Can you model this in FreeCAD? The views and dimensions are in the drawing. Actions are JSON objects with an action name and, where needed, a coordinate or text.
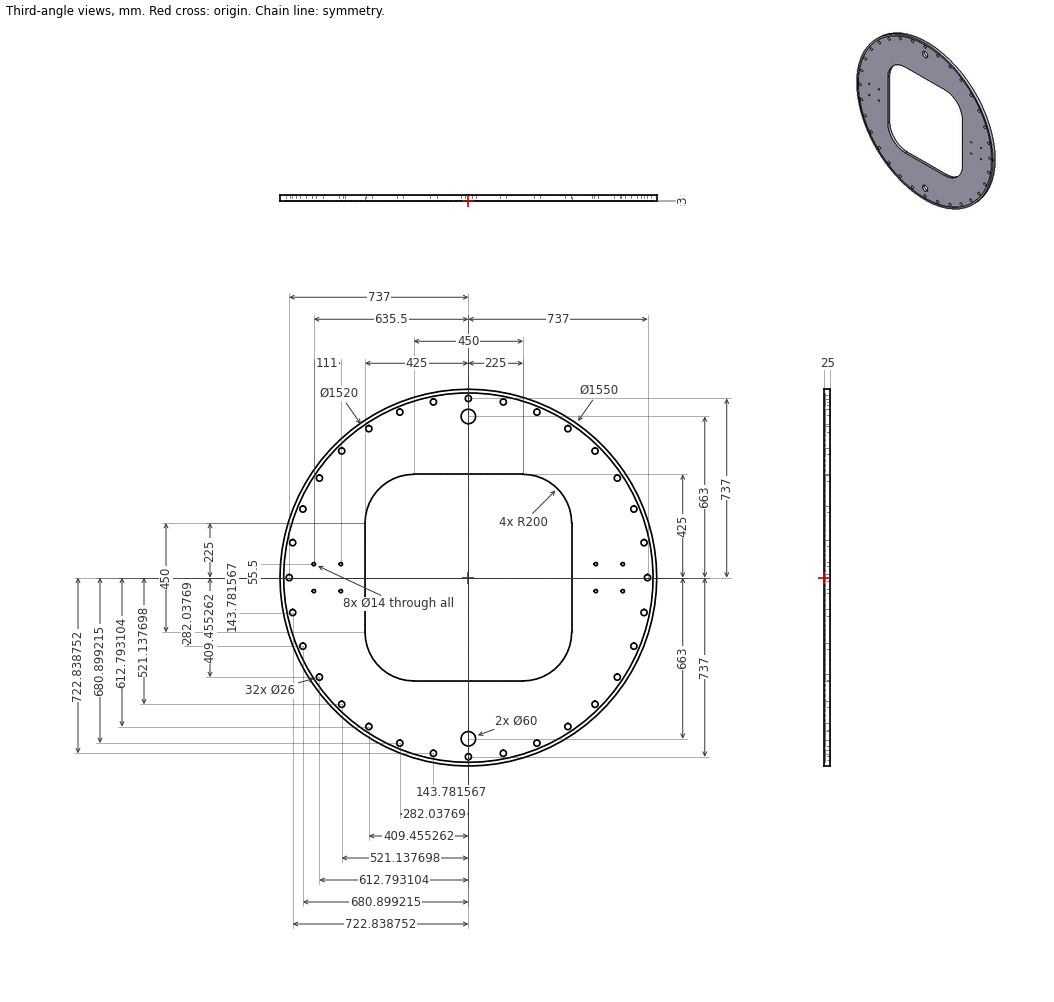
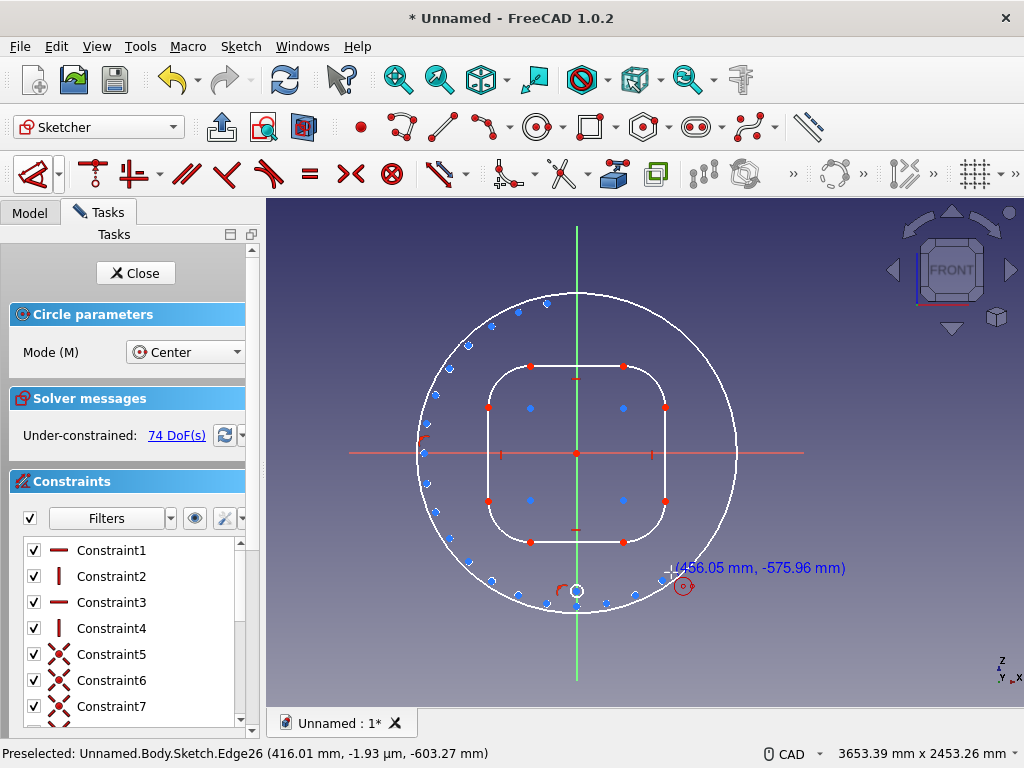
{"action": "scroll", "coordinate": [685, 561], "scroll_direction": "up", "scroll_amount": 4}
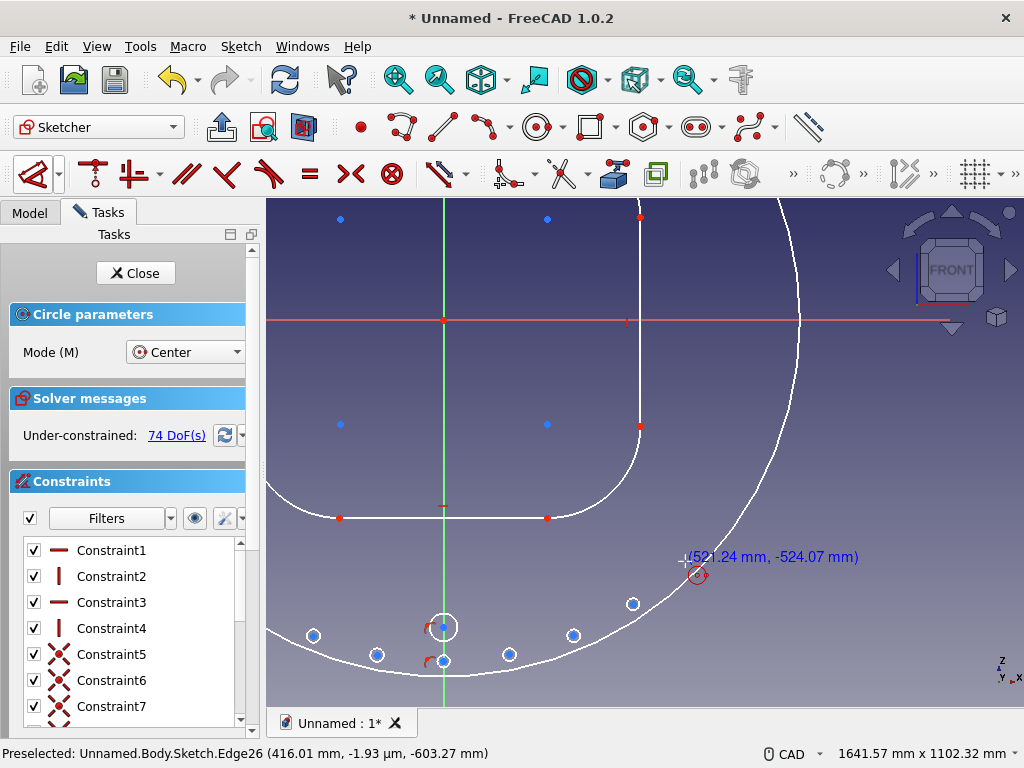
{"action": "left_click", "coordinate": [684, 561]}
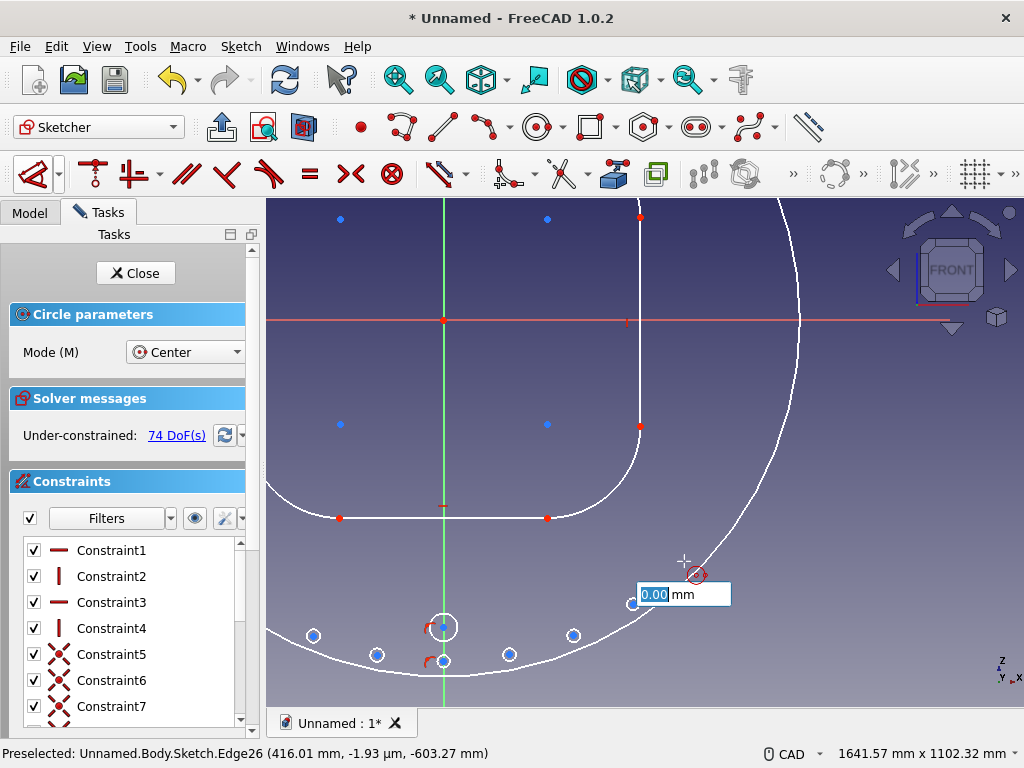
{"action": "scroll", "coordinate": [689, 557], "scroll_direction": "up", "scroll_amount": 5}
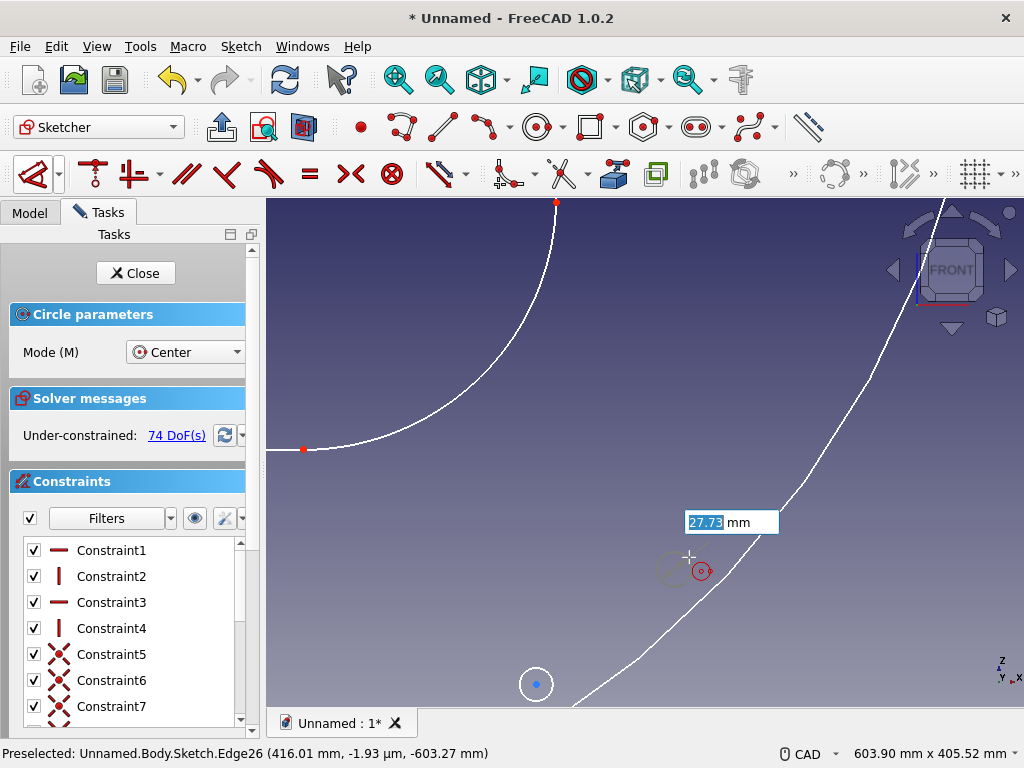
{"action": "left_click", "coordinate": [687, 555]}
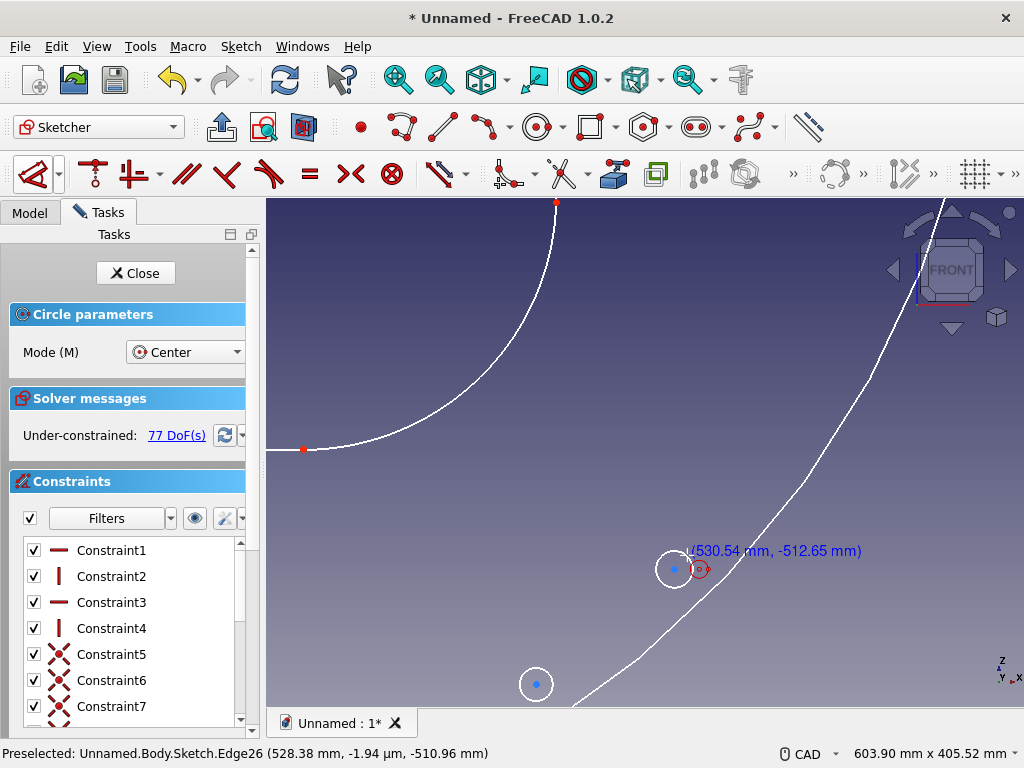
{"action": "scroll", "coordinate": [790, 426], "scroll_direction": "up", "scroll_amount": 2}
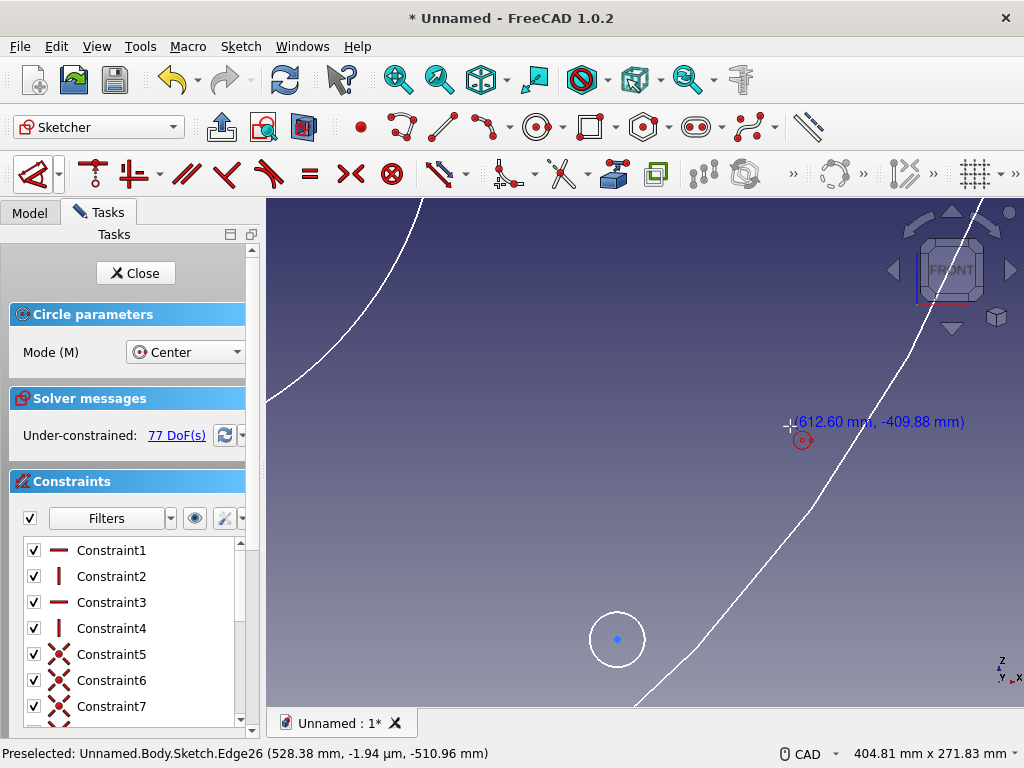
{"action": "scroll", "coordinate": [693, 551], "scroll_direction": "down", "scroll_amount": 11}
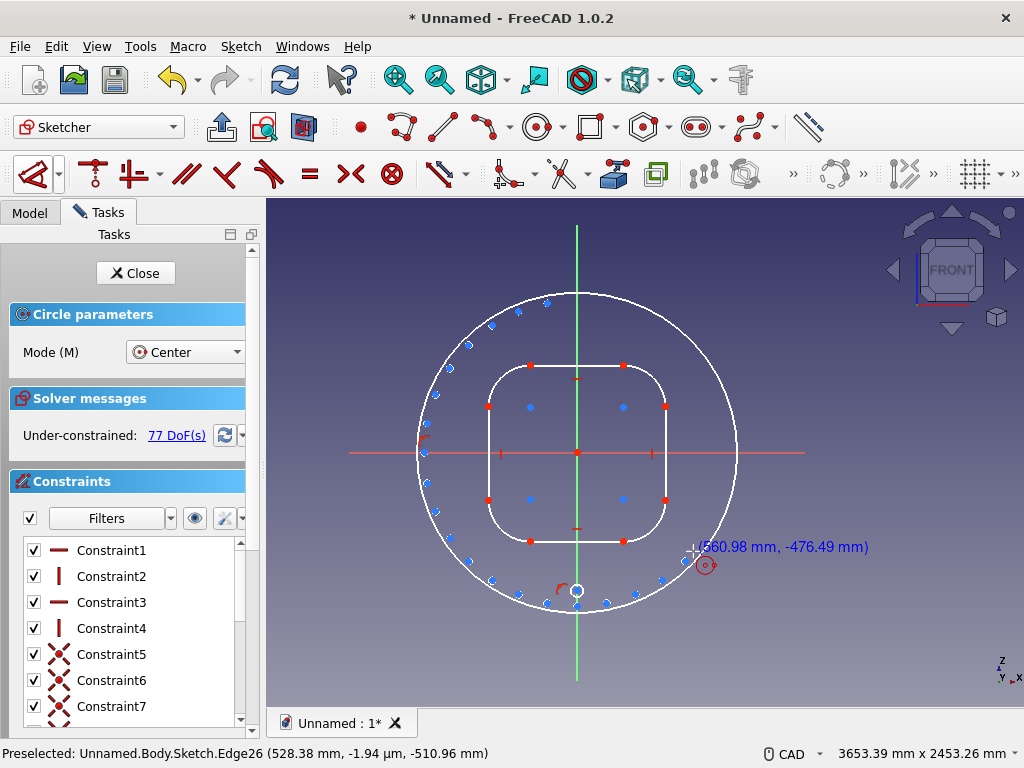
{"action": "scroll", "coordinate": [704, 538], "scroll_direction": "up", "scroll_amount": 4}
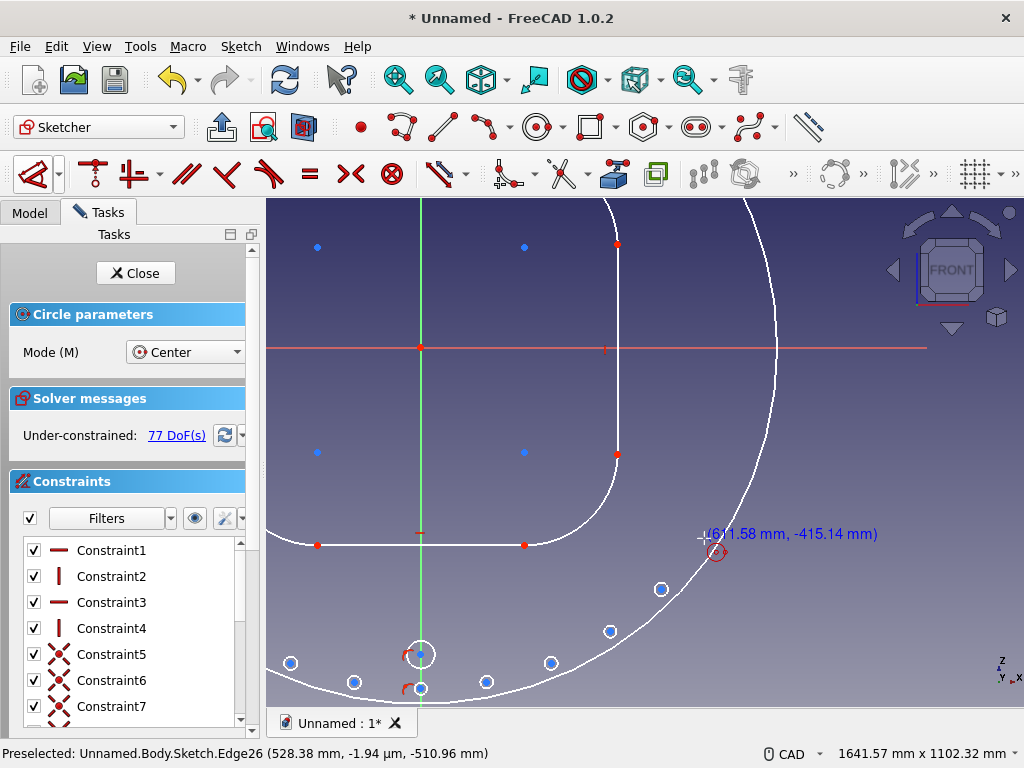
{"action": "left_click", "coordinate": [704, 537]}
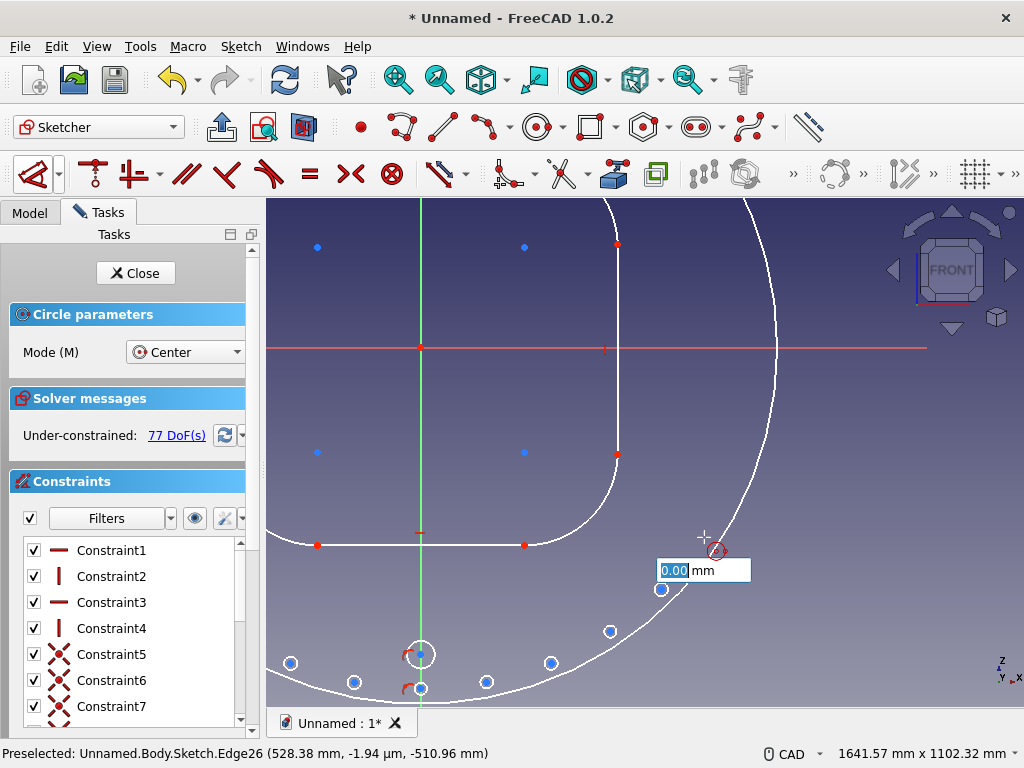
{"action": "scroll", "coordinate": [708, 533], "scroll_direction": "up", "scroll_amount": 5}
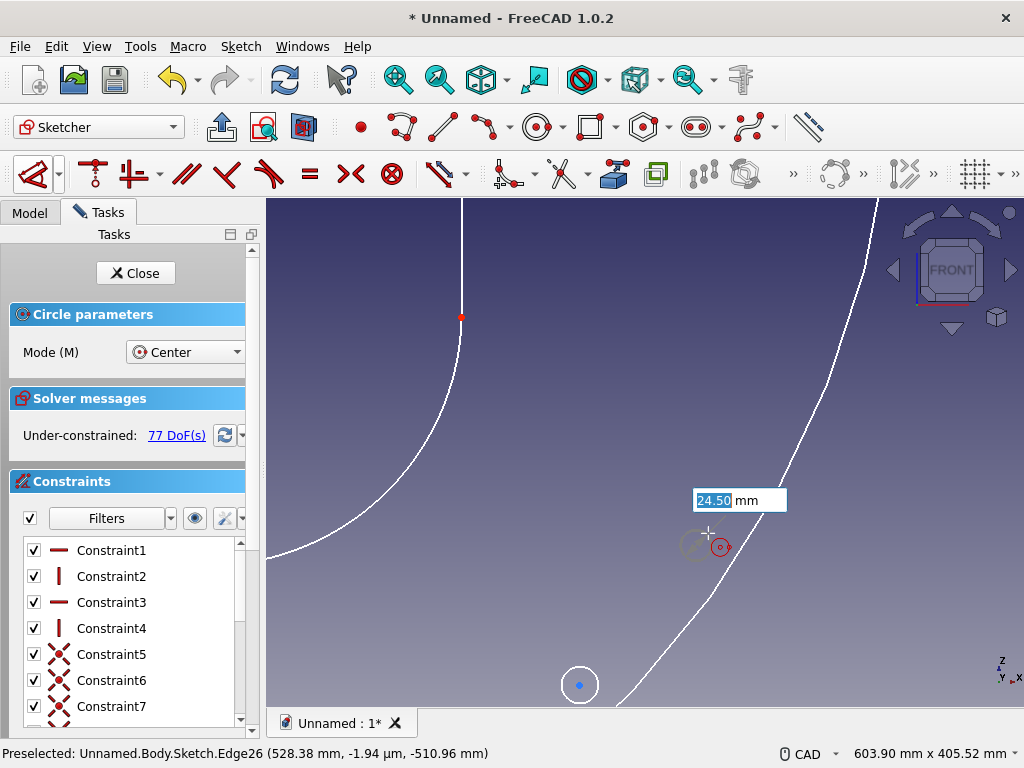
{"action": "left_click", "coordinate": [707, 531]}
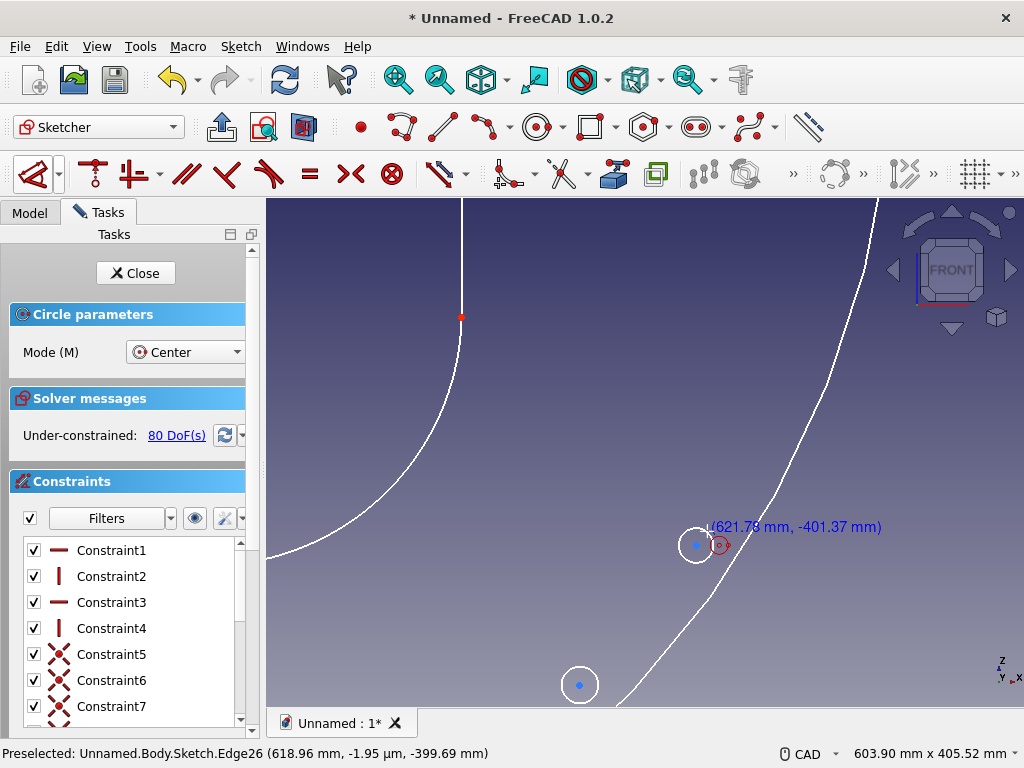
{"action": "scroll", "coordinate": [781, 382], "scroll_direction": "up", "scroll_amount": 2}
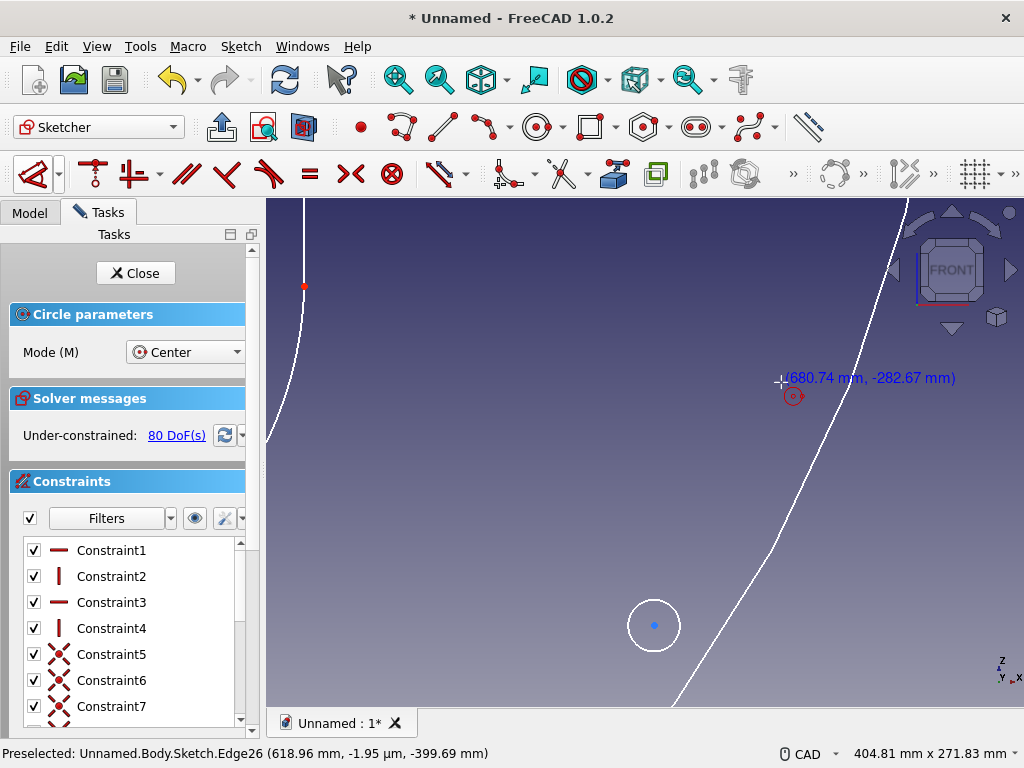
{"action": "scroll", "coordinate": [710, 527], "scroll_direction": "down", "scroll_amount": 11}